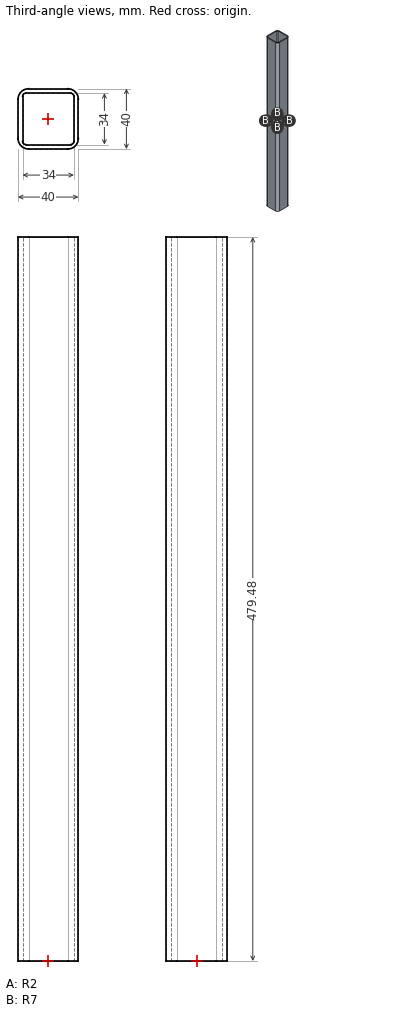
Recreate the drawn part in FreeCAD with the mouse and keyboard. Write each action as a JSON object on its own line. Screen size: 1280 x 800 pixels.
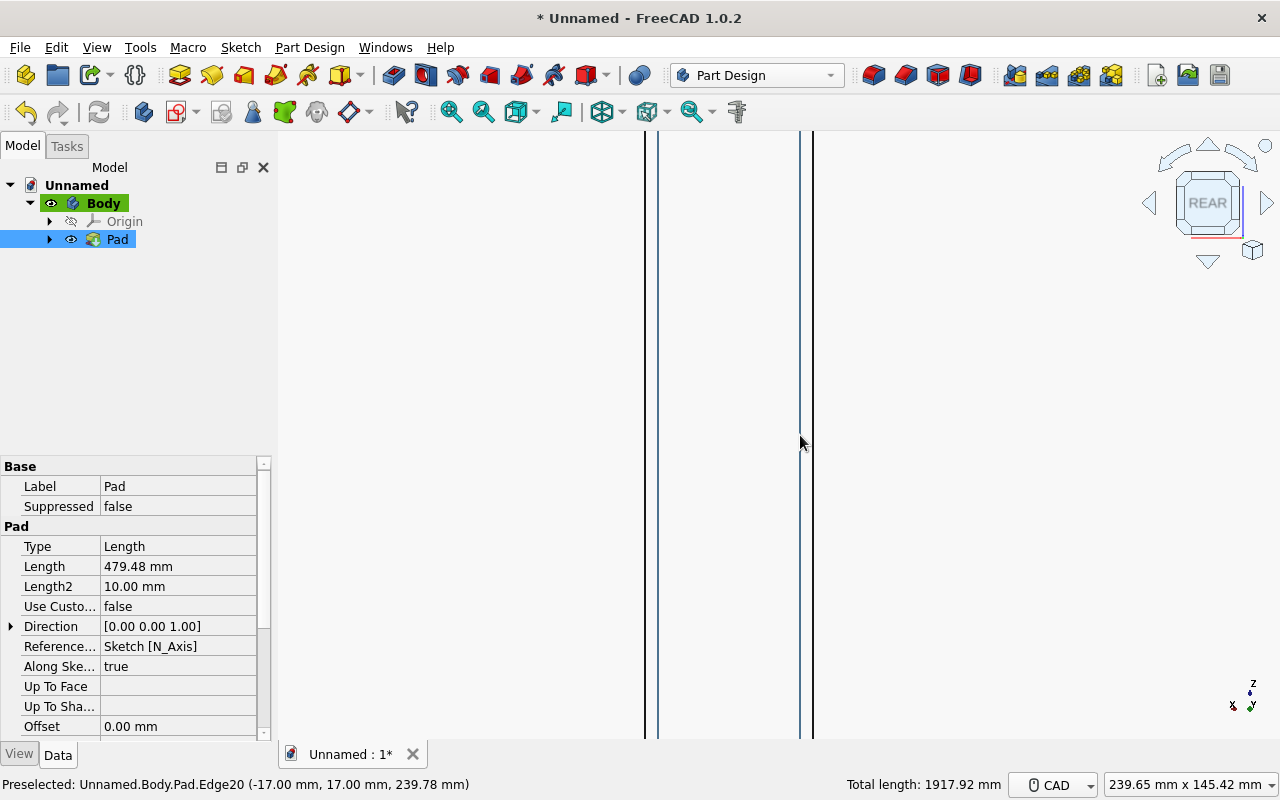
{"action": "key", "text": "v 1"}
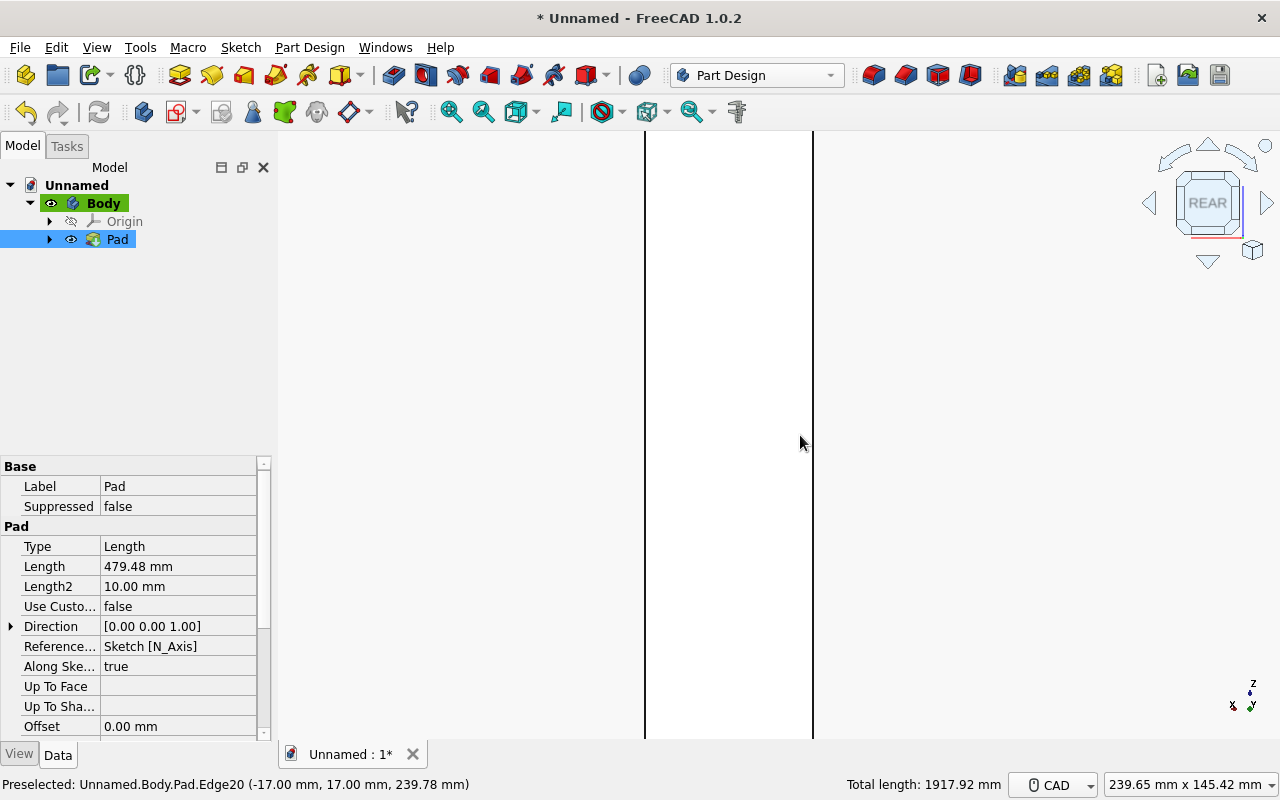
{"action": "left_click", "coordinate": [874, 76]}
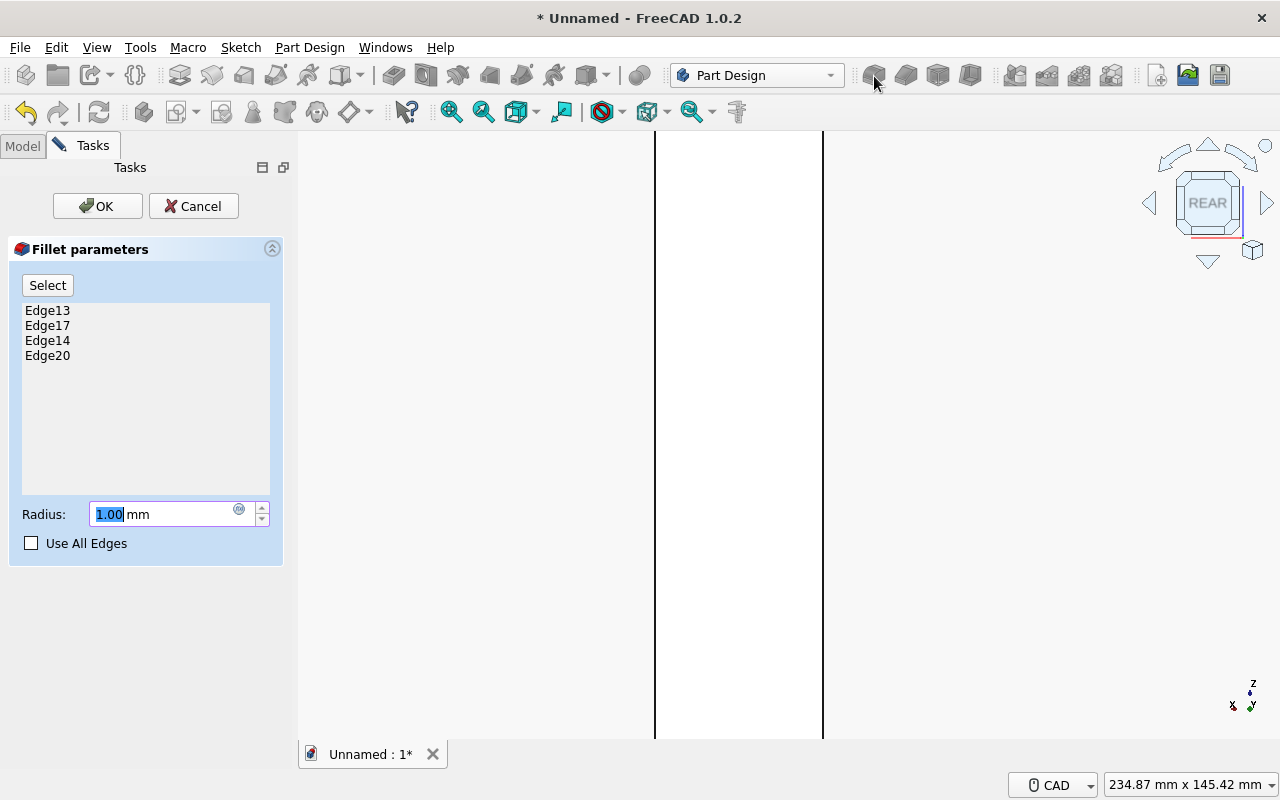
{"action": "type", "text": "2"}
{"action": "key", "text": "Tab"}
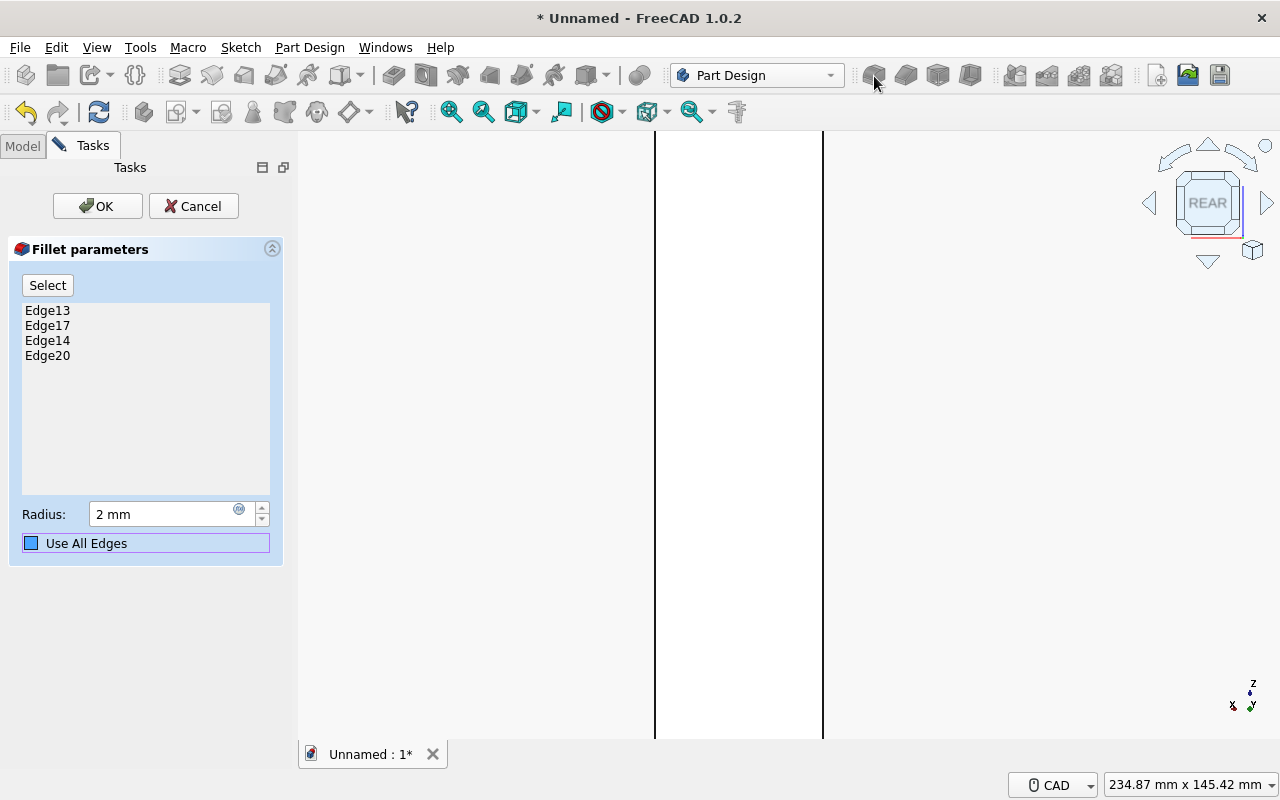
{"action": "left_click", "coordinate": [98, 206]}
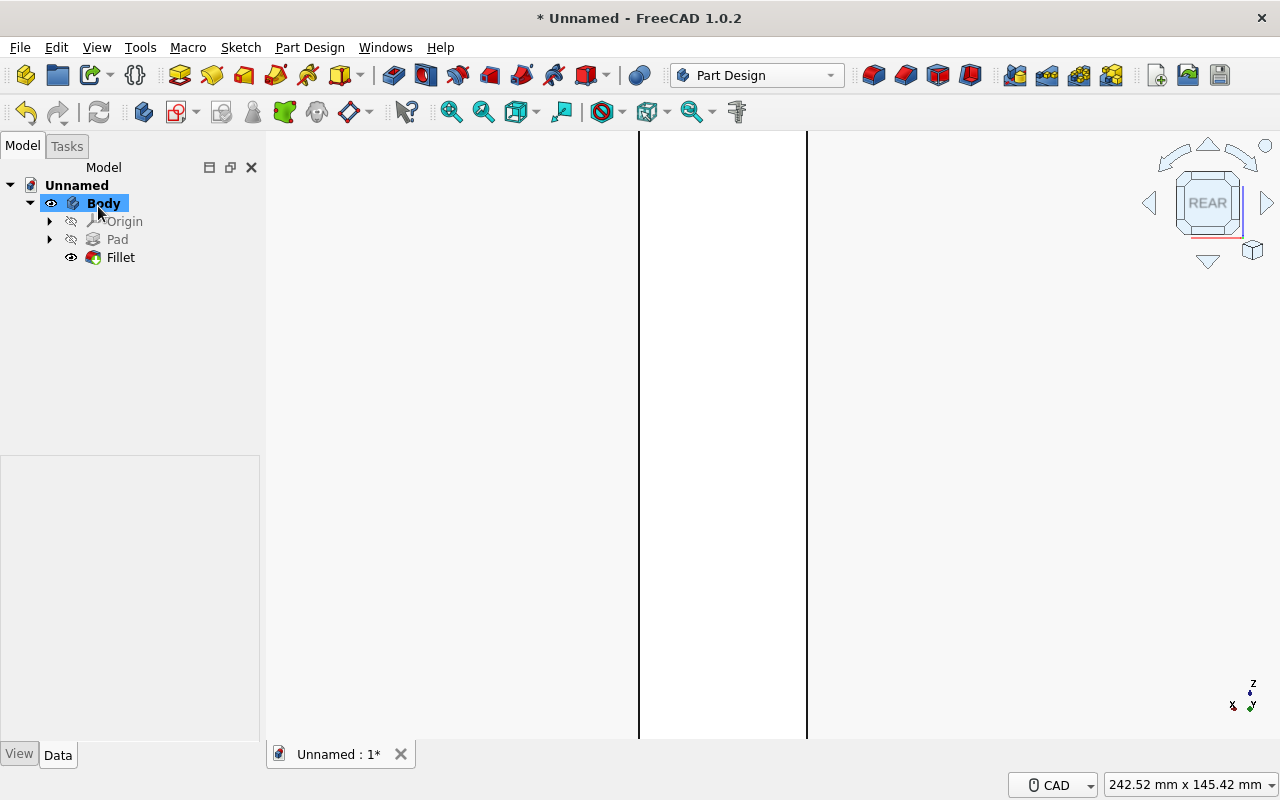
{"action": "key", "text": "v f"}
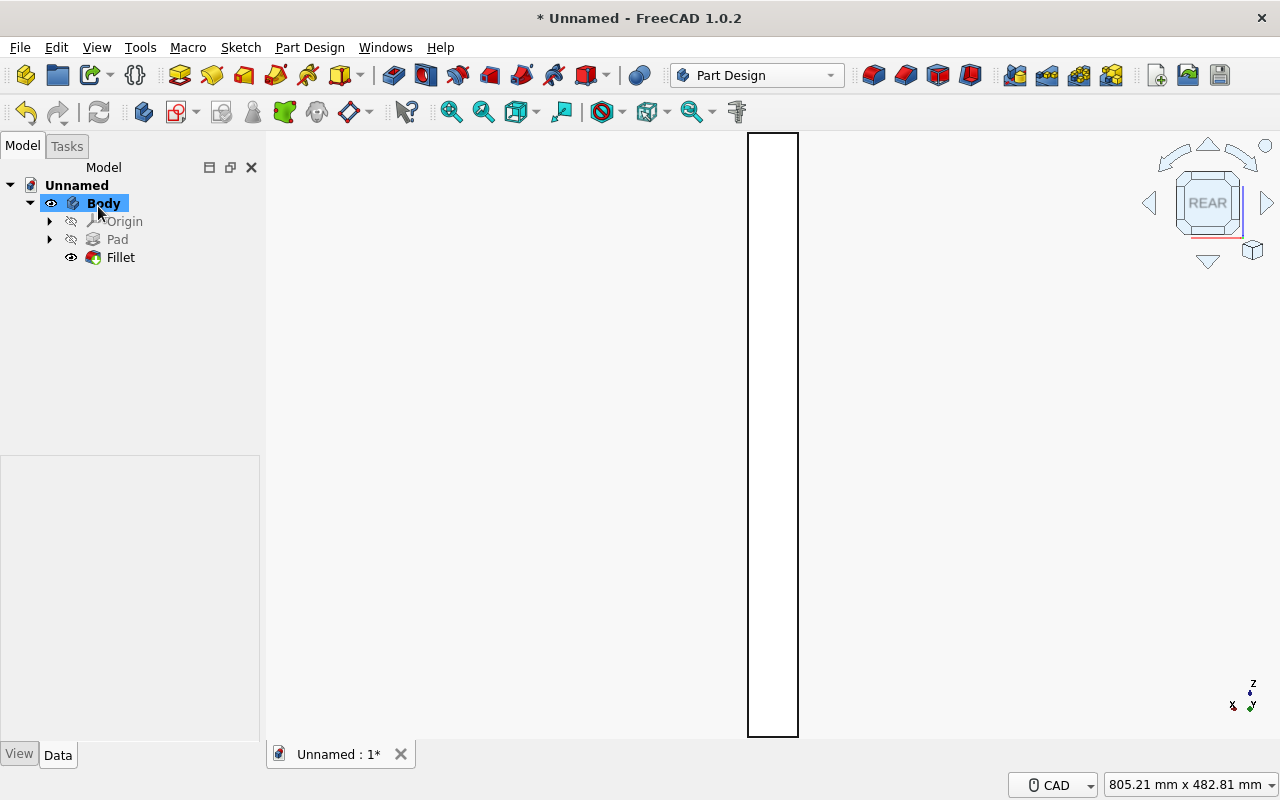
{"action": "left_click", "coordinate": [798, 434]}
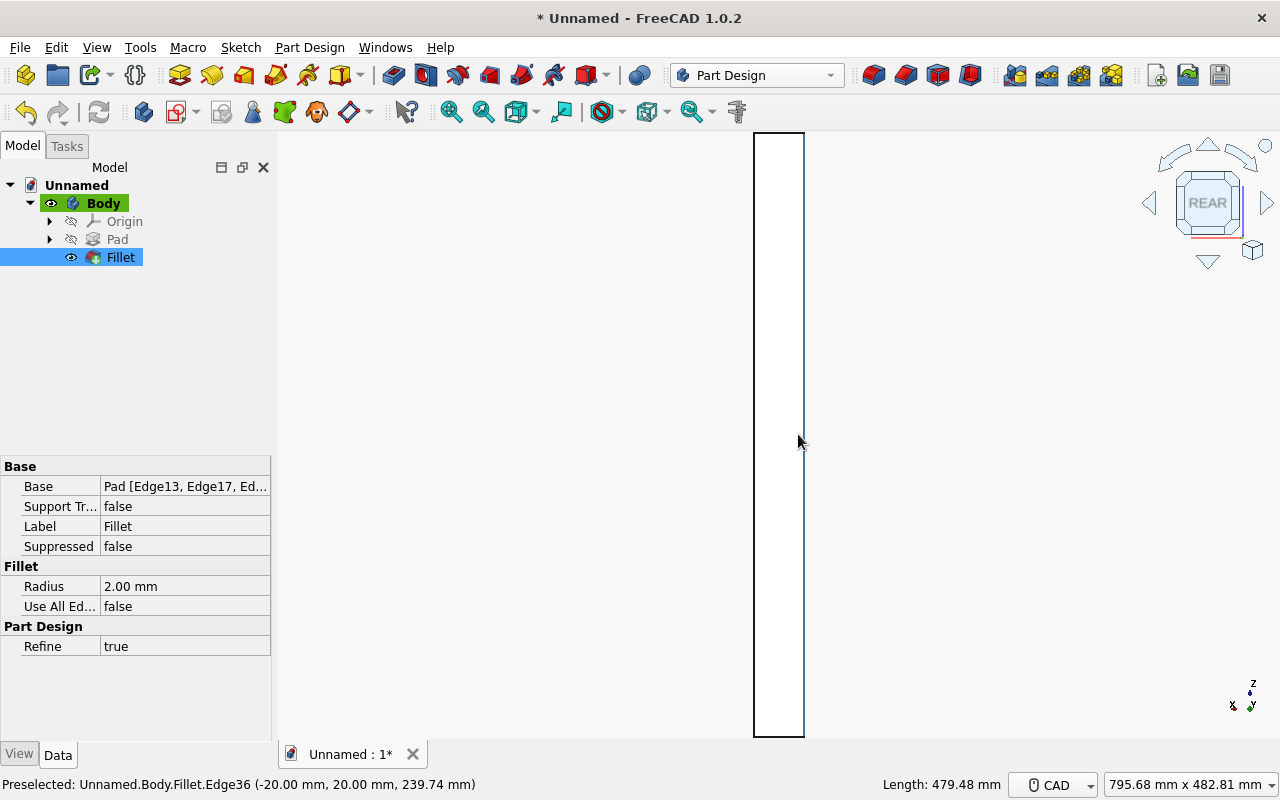
{"action": "left_click", "coordinate": [754, 434], "text": "ctrl"}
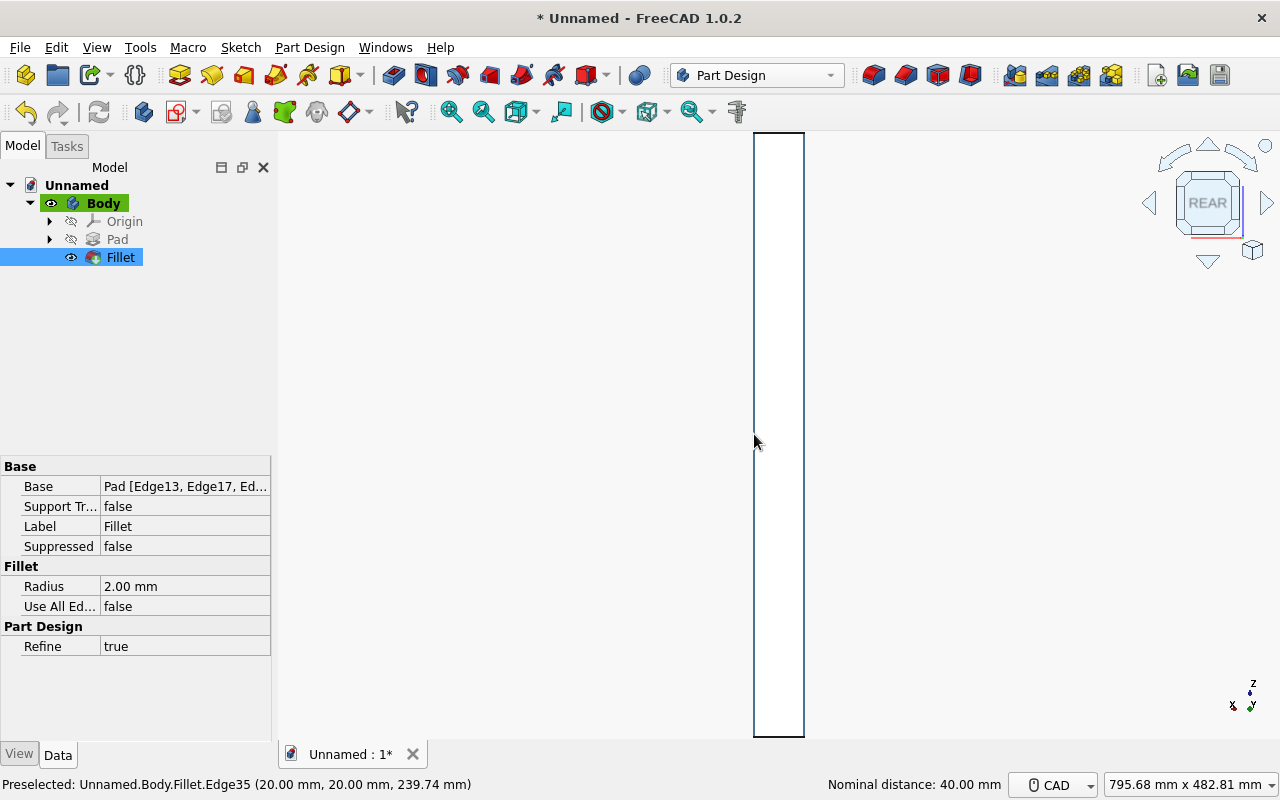
{"action": "key", "text": "0"}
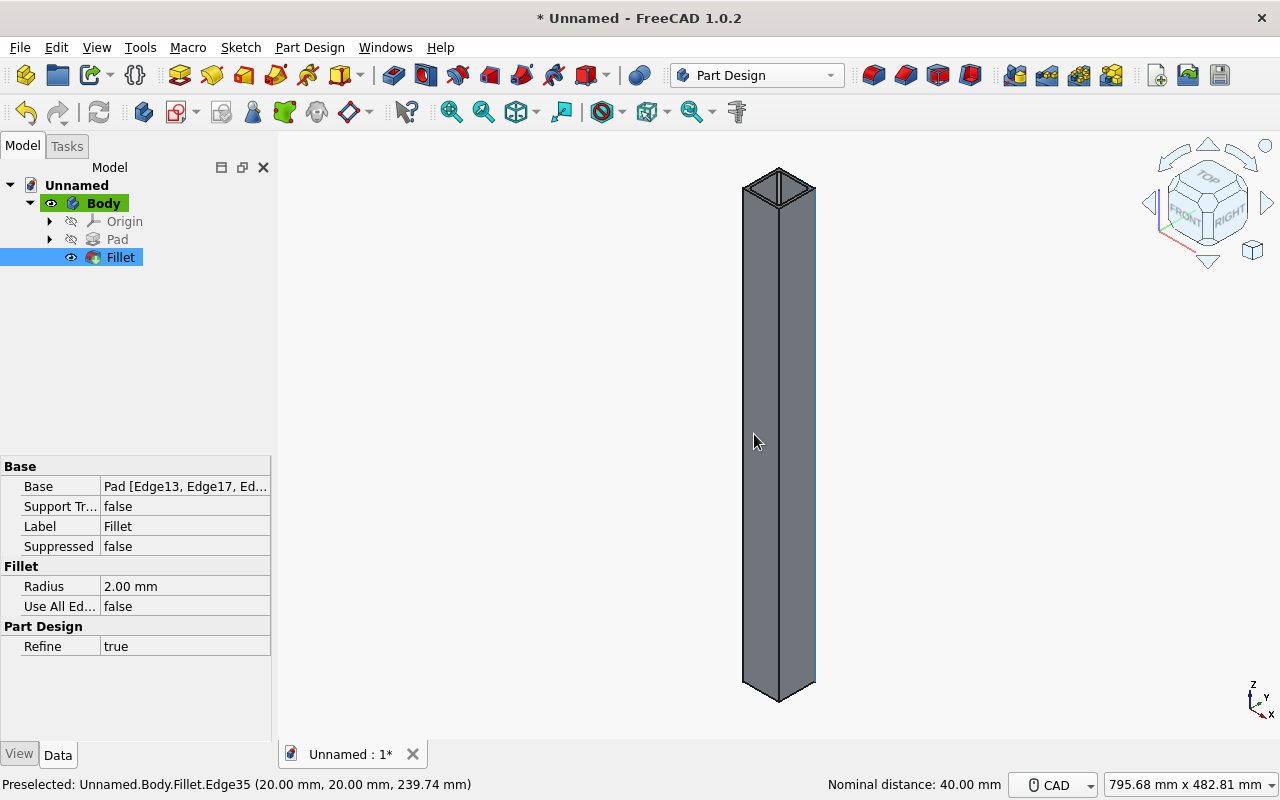
{"action": "left_click", "coordinate": [779, 455], "text": "ctrl"}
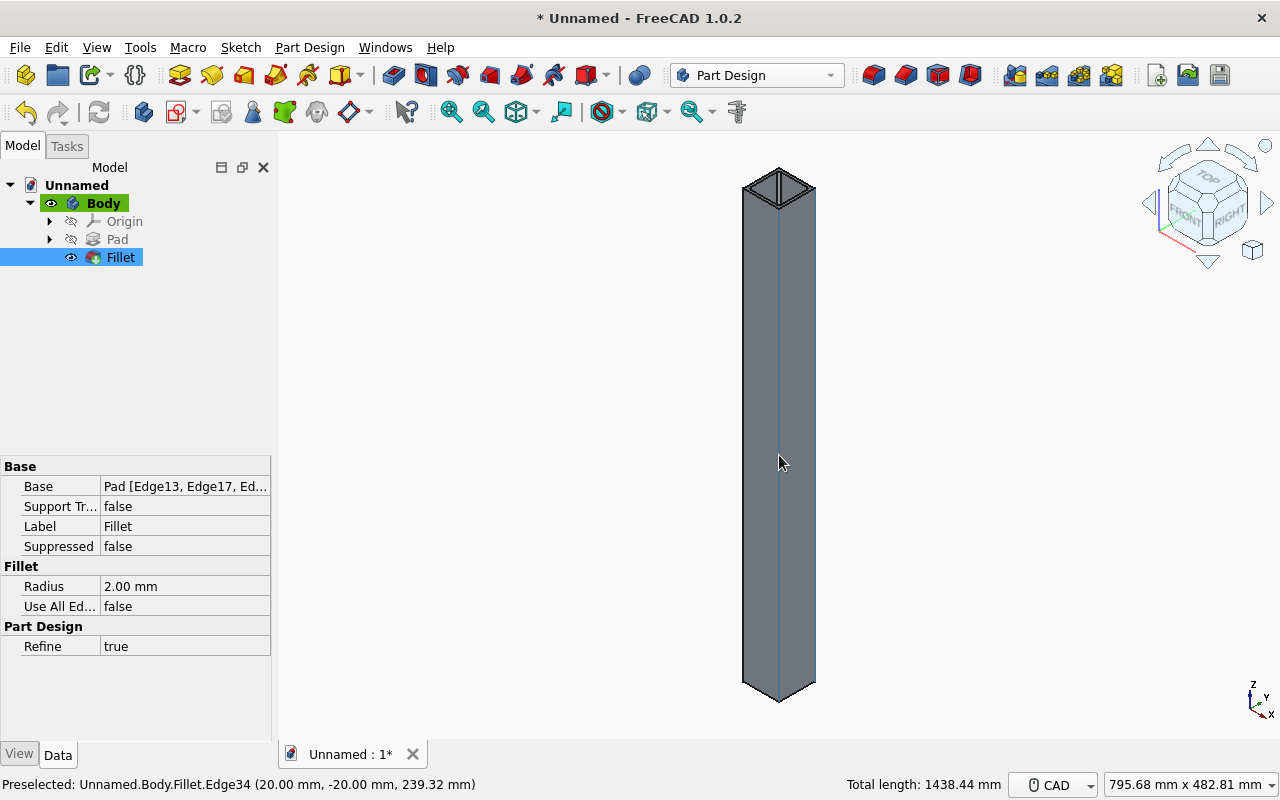
{"action": "key", "text": "2"}